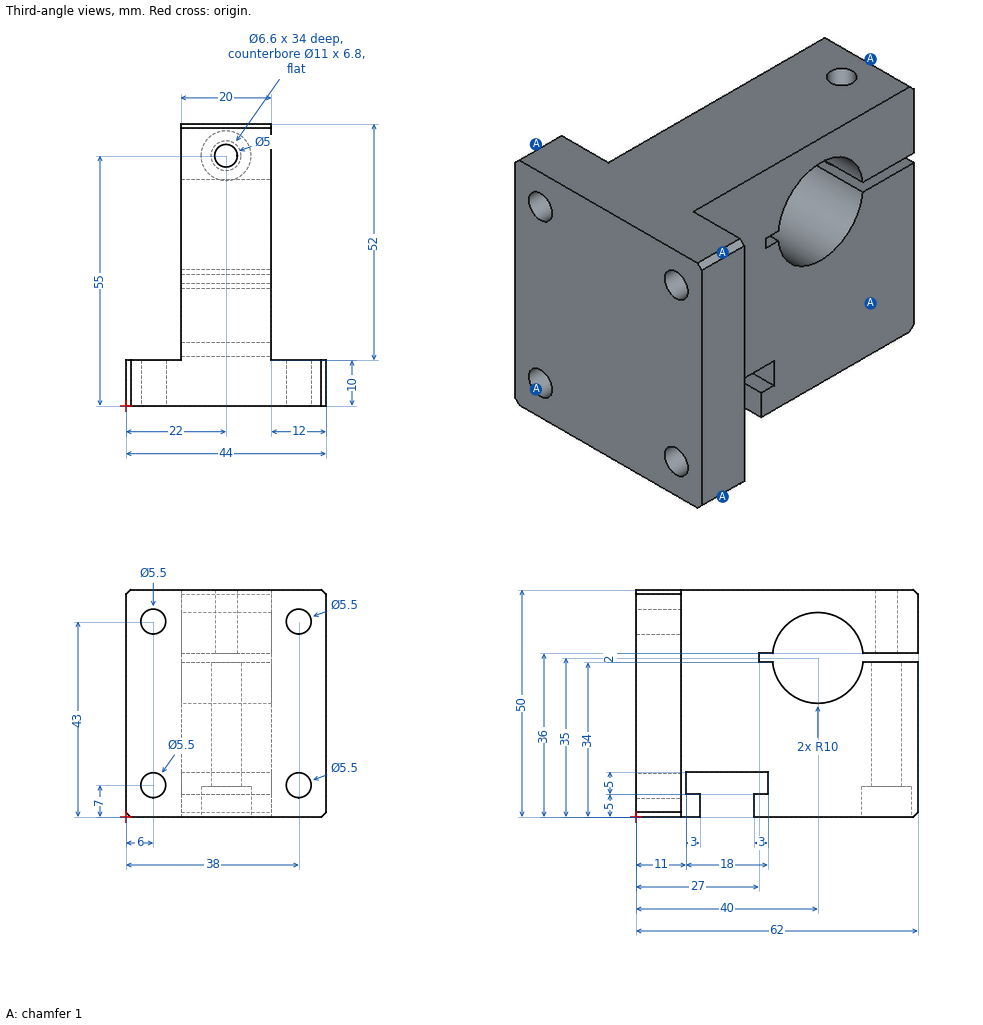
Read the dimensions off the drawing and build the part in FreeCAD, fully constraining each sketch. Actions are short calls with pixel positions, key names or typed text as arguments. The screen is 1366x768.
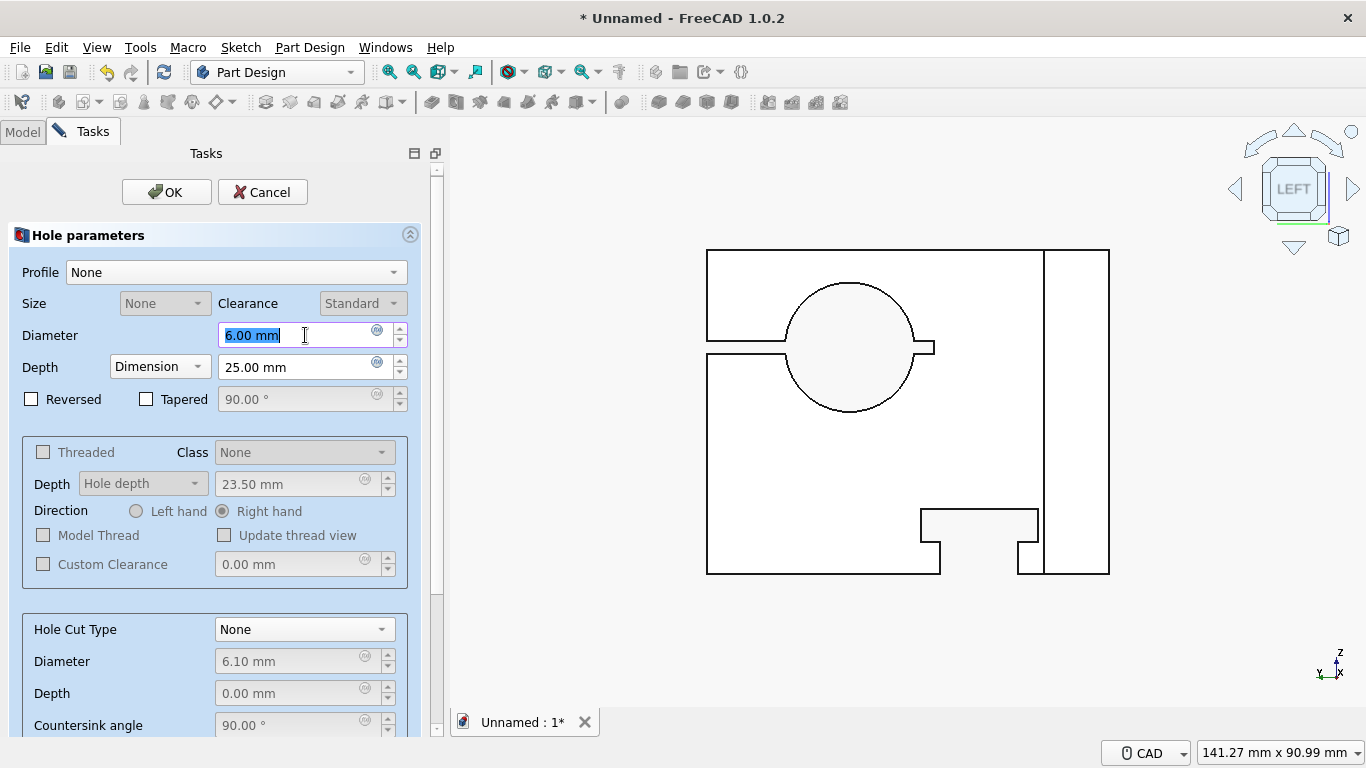
text(6.6)
key(Tab)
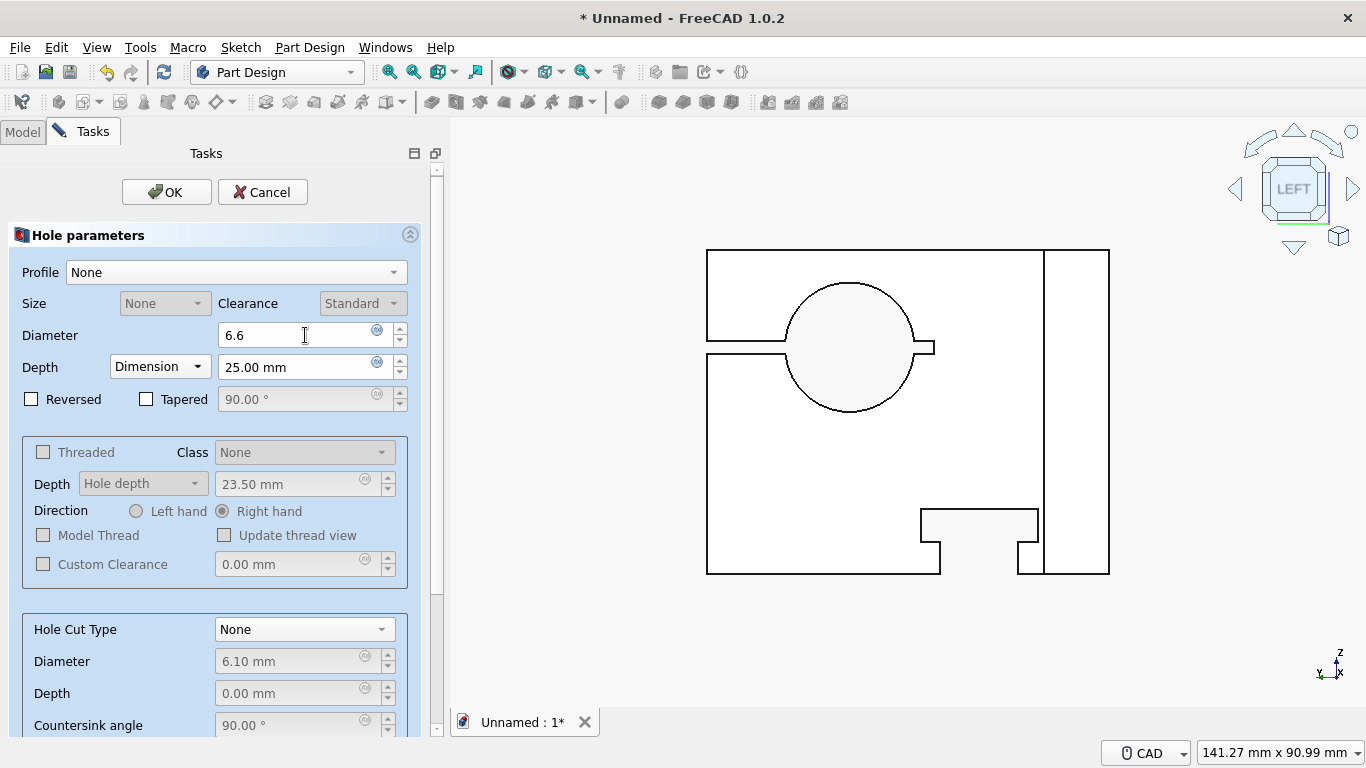
triple_click(305, 367)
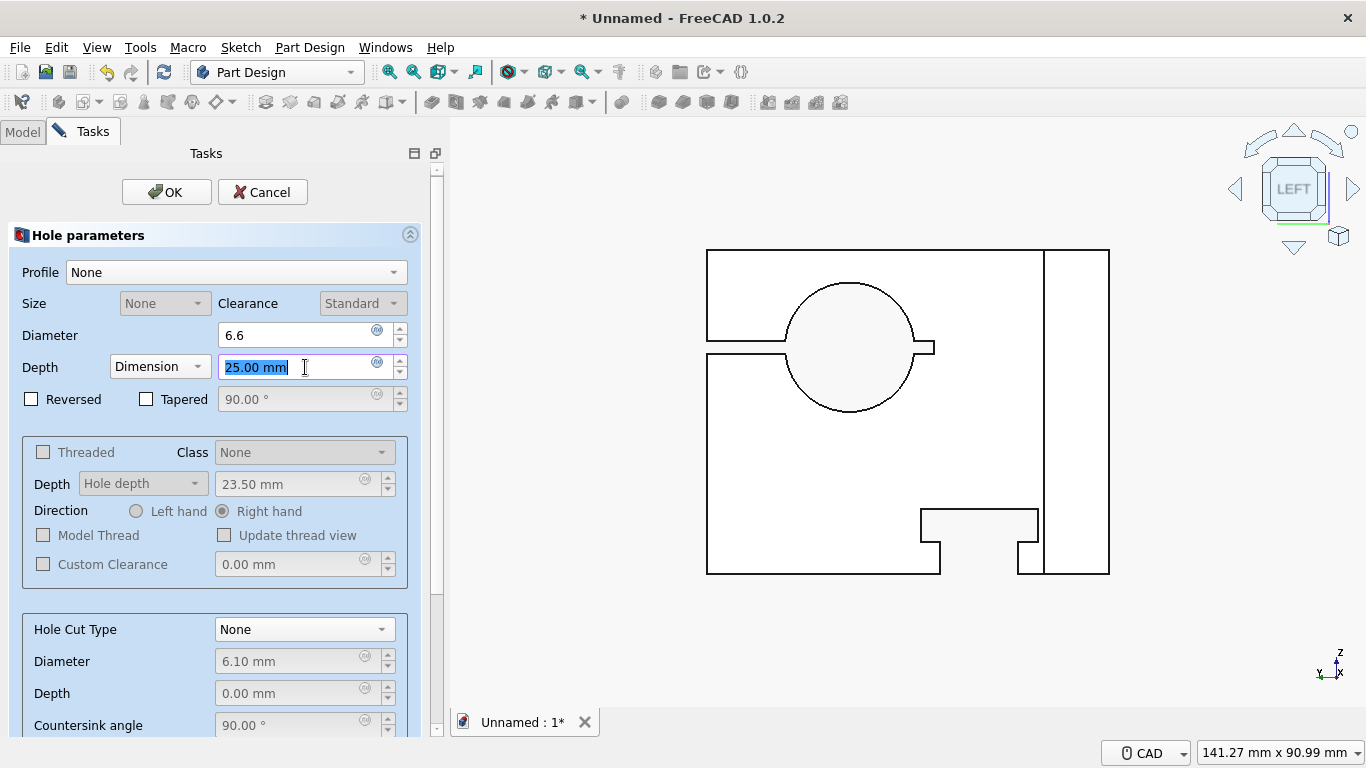
text(34)
key(Tab)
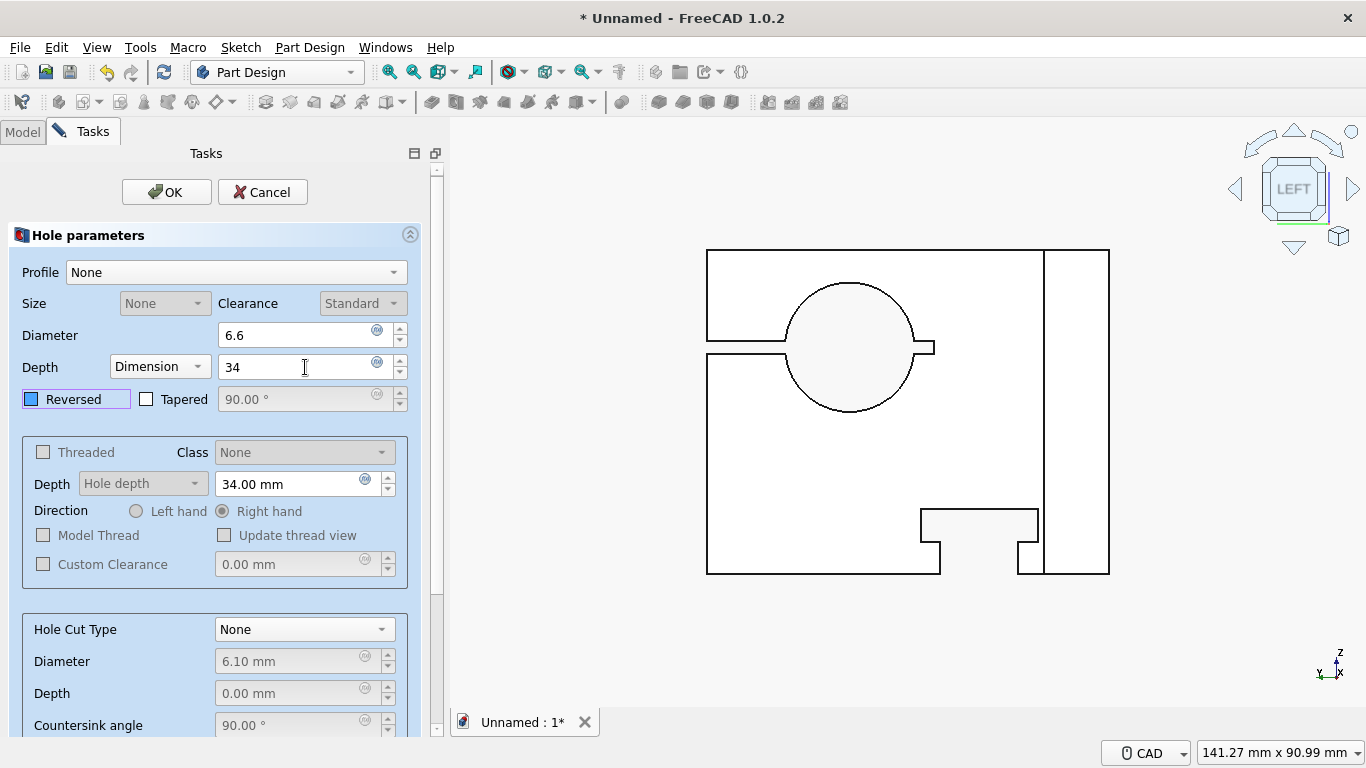
click(30, 399)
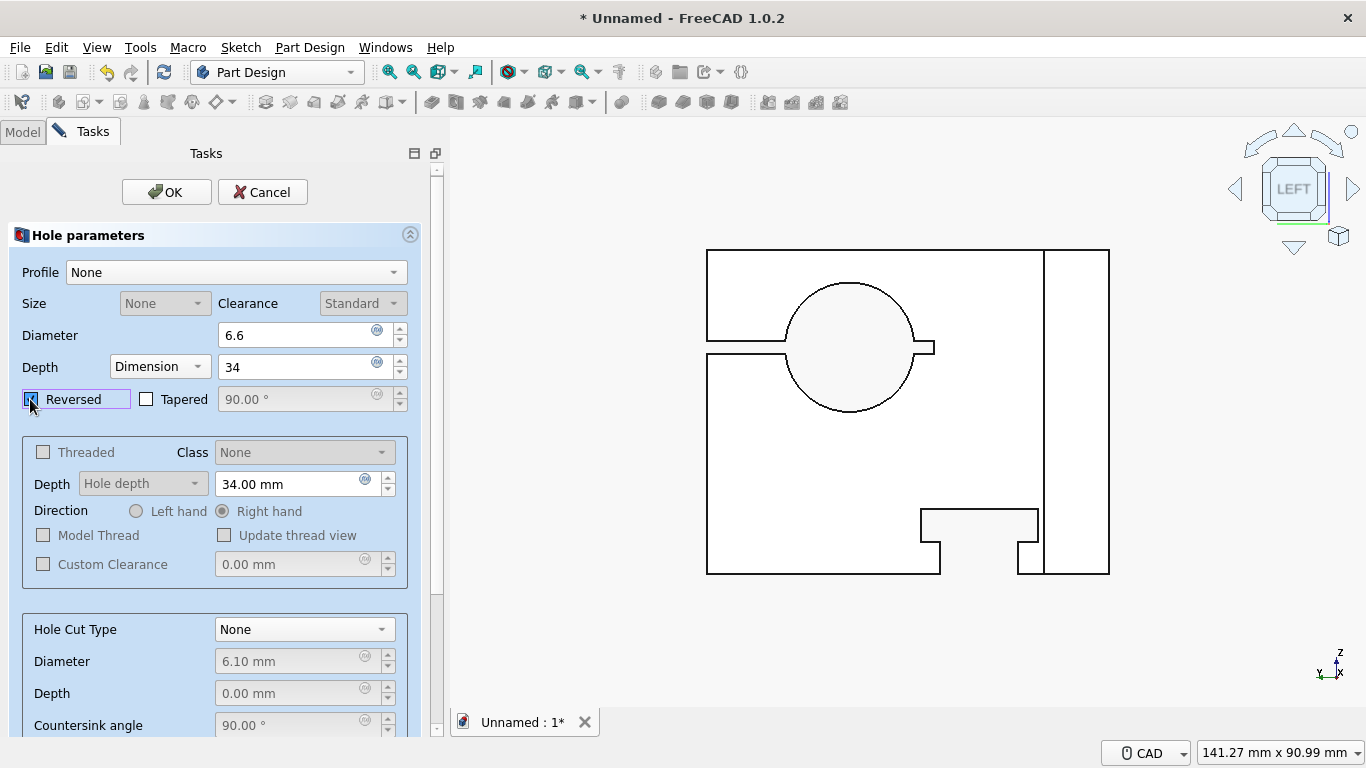
click(306, 630)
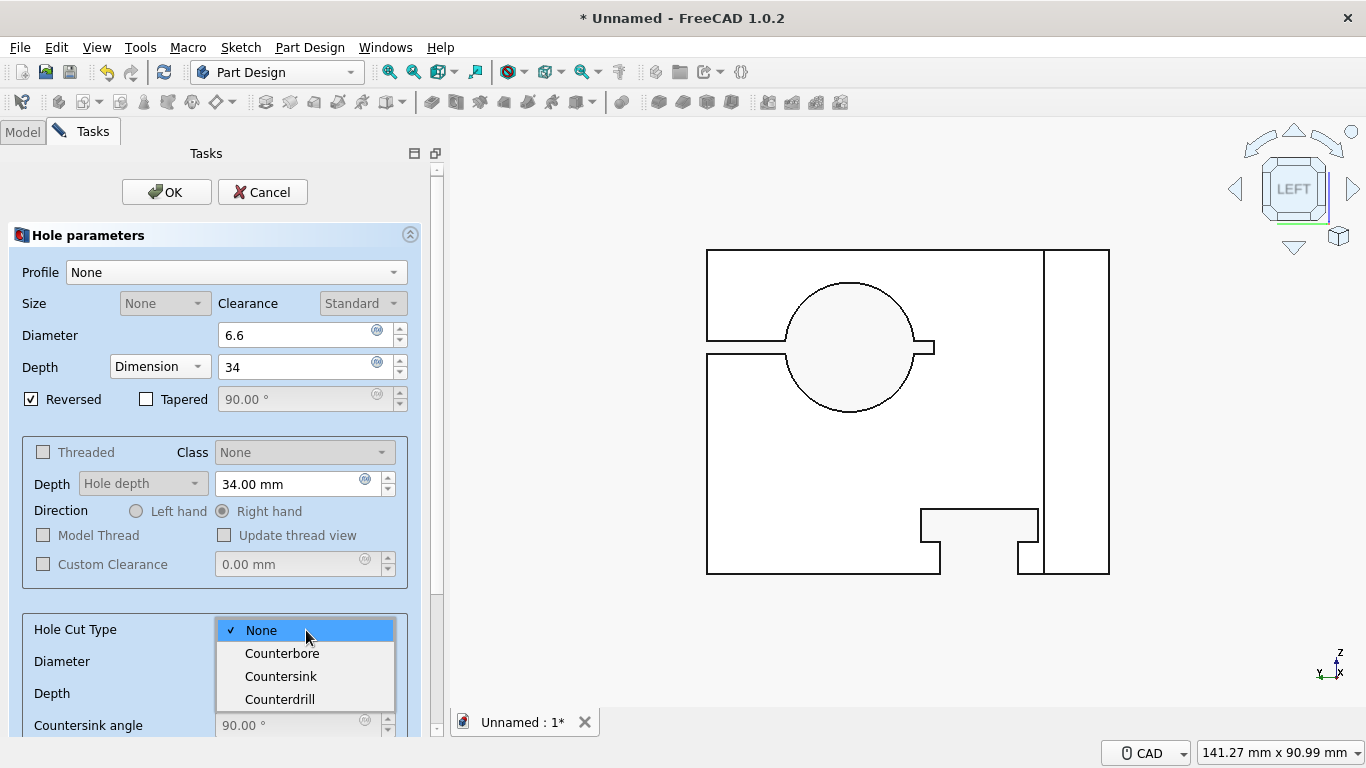
click(304, 654)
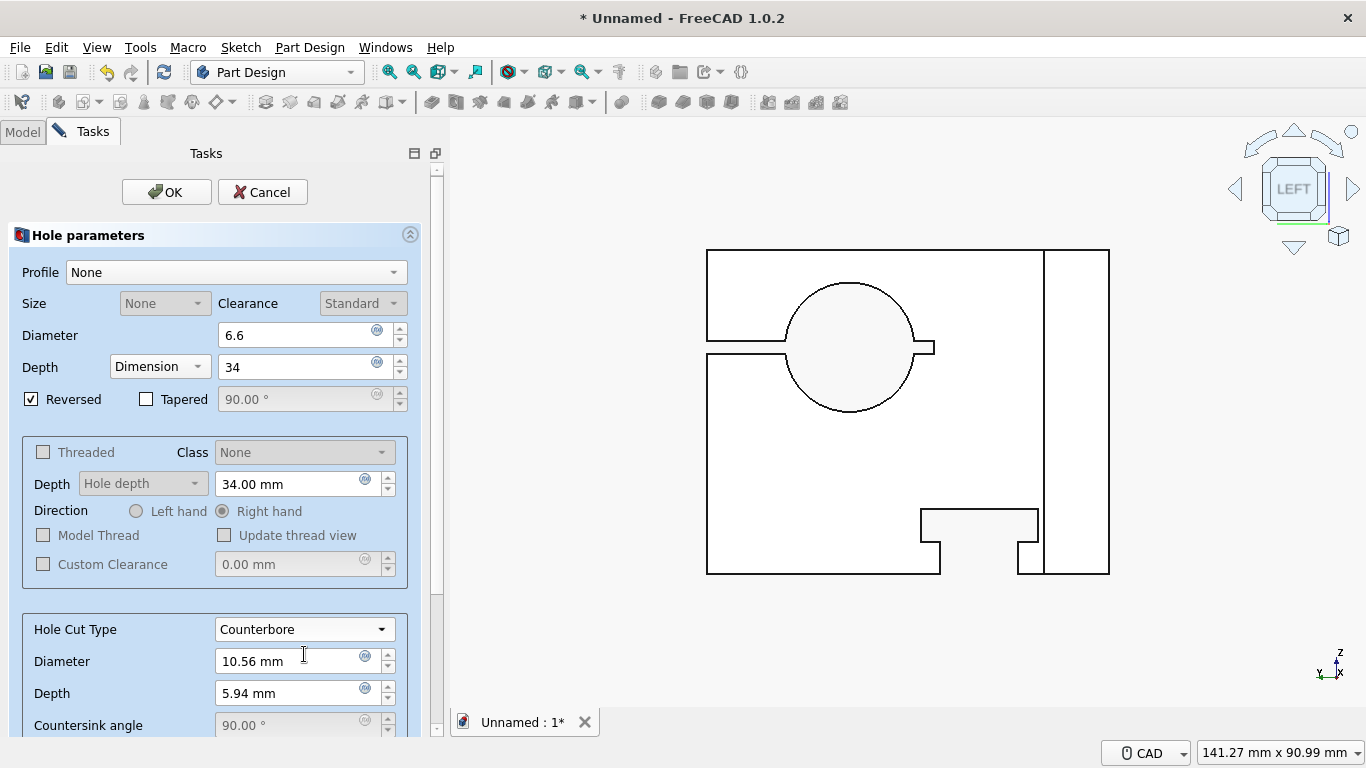
triple_click(298, 661)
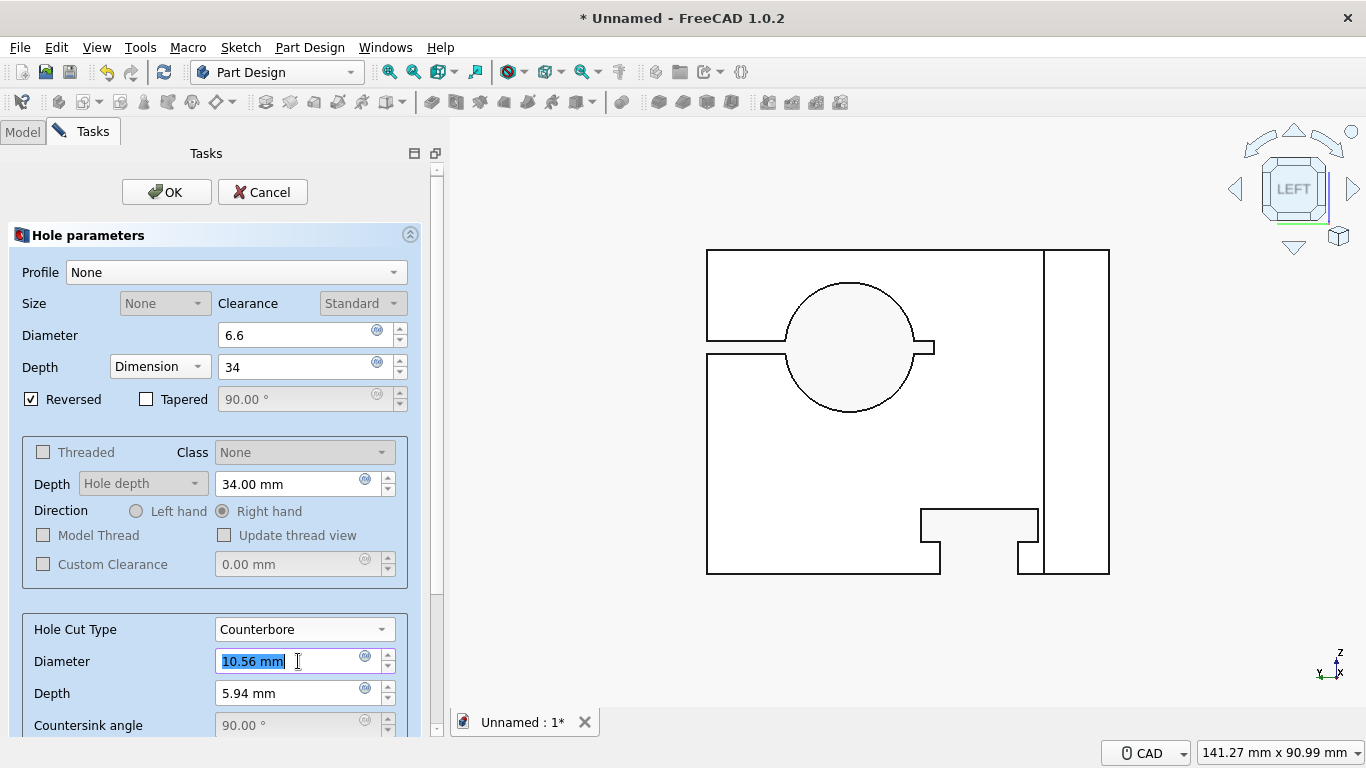
text(11)
key(Tab)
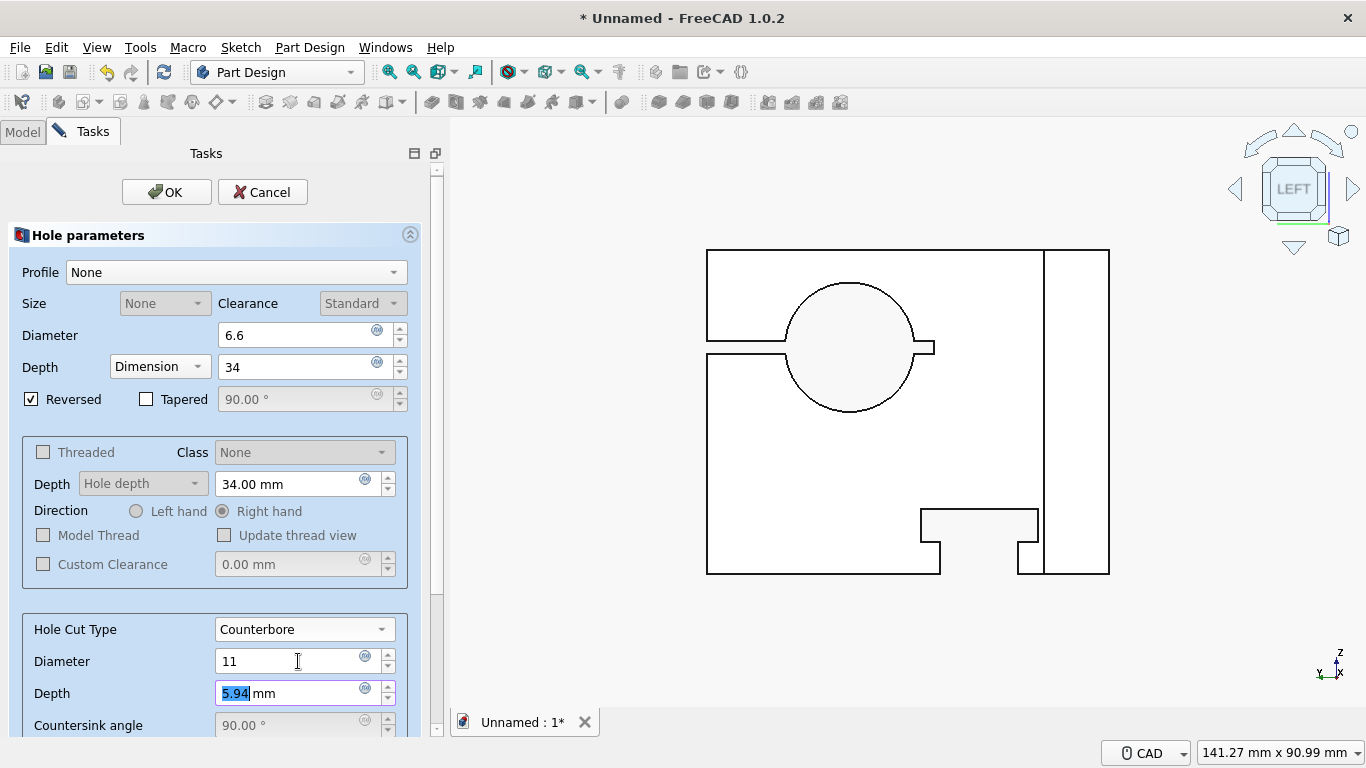
text(6.8)
key(Tab)